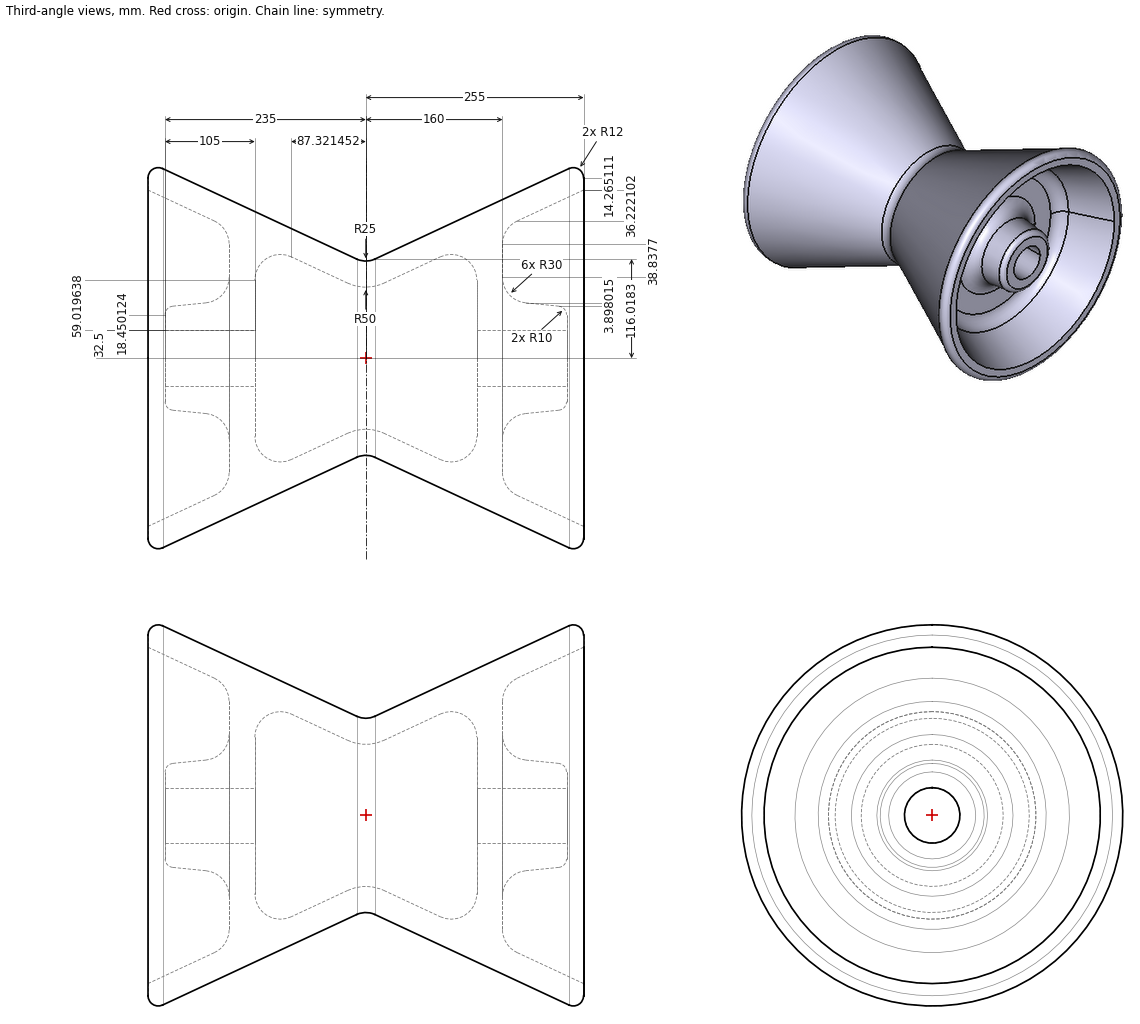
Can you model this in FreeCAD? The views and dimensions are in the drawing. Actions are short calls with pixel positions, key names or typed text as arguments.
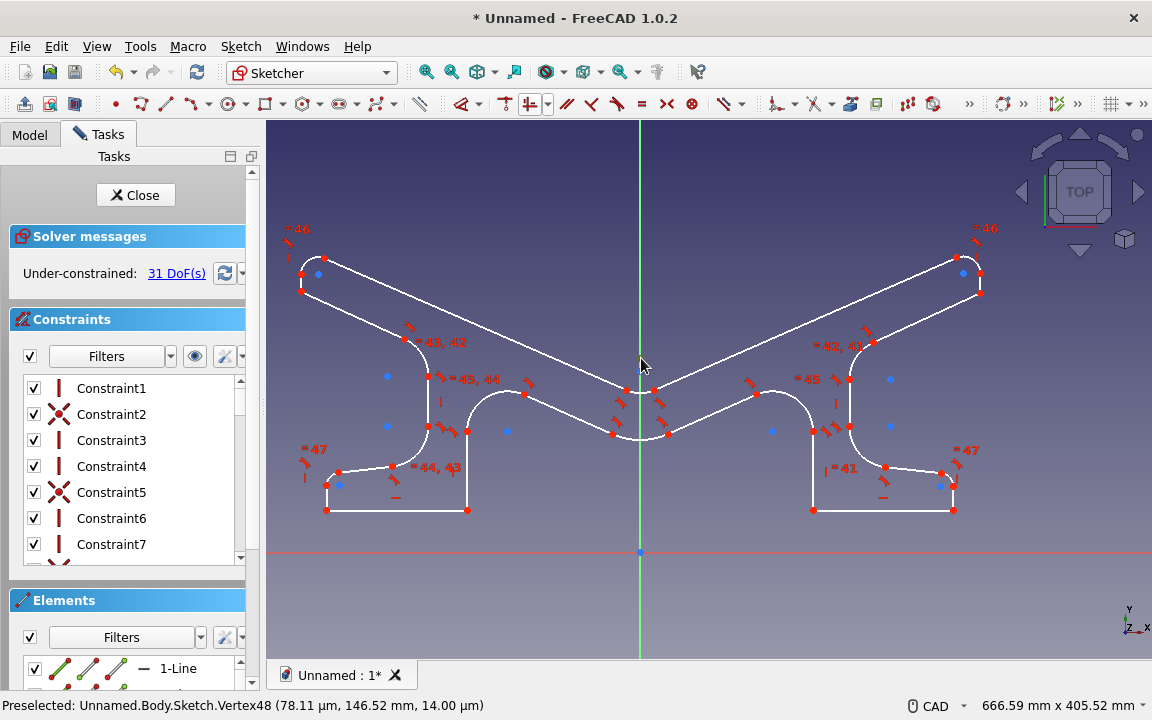
click(640, 596)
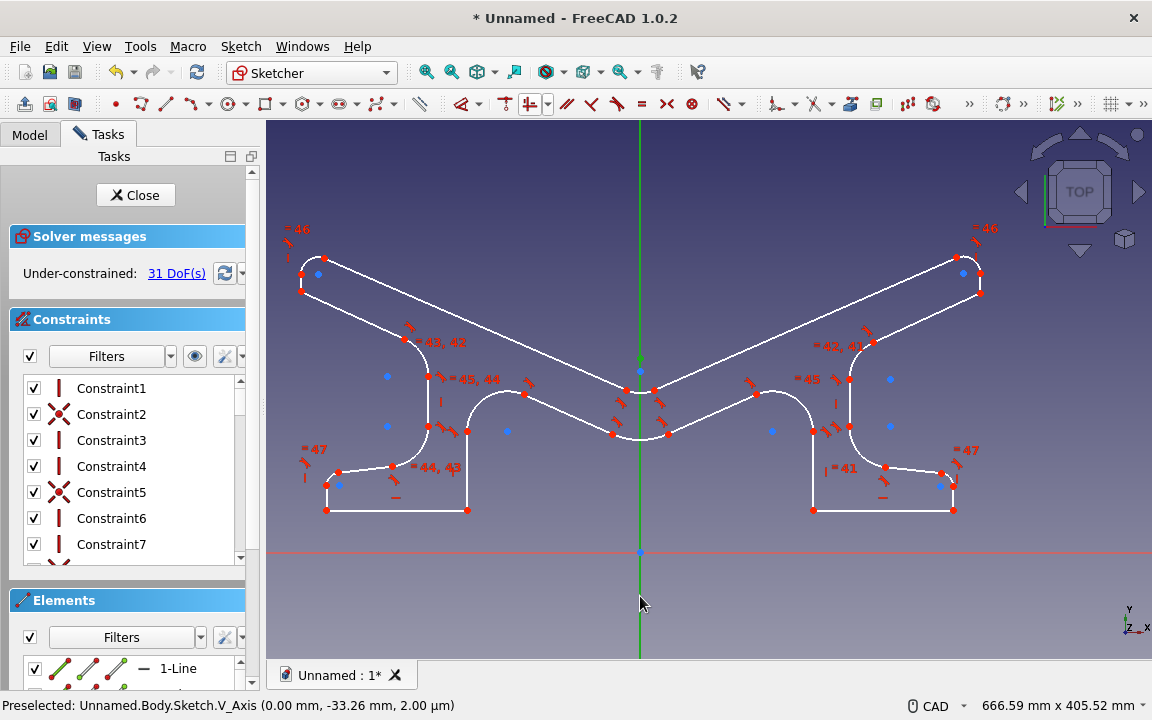
key(c)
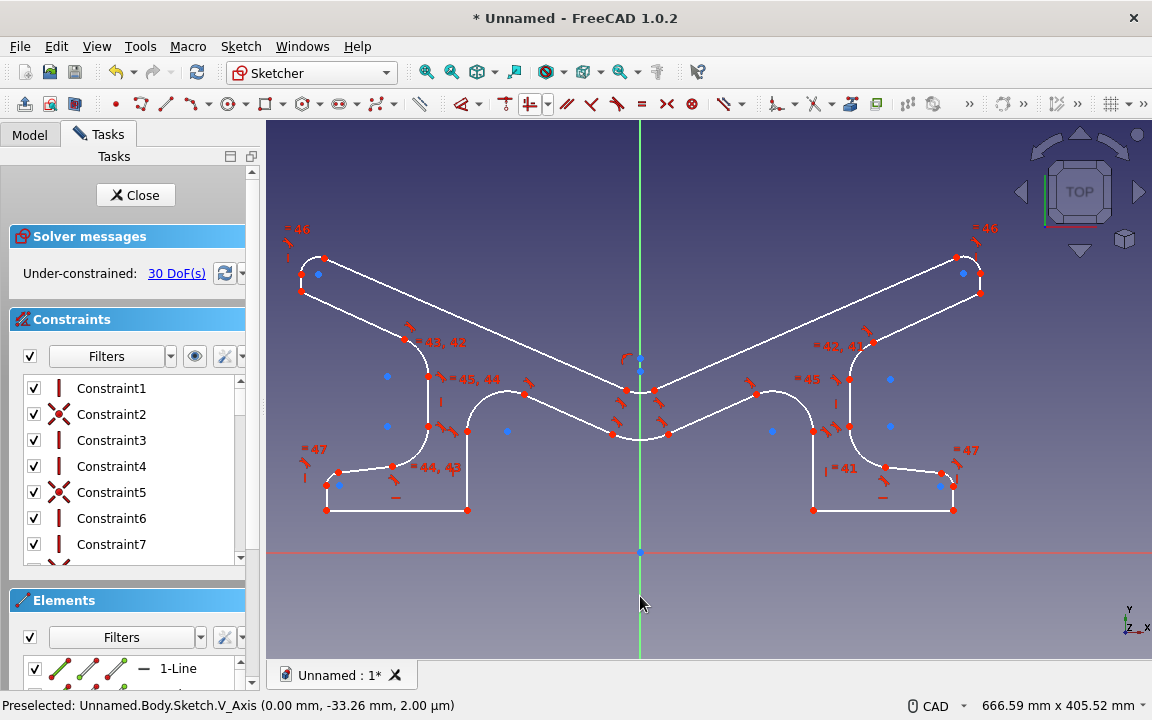
click(640, 371)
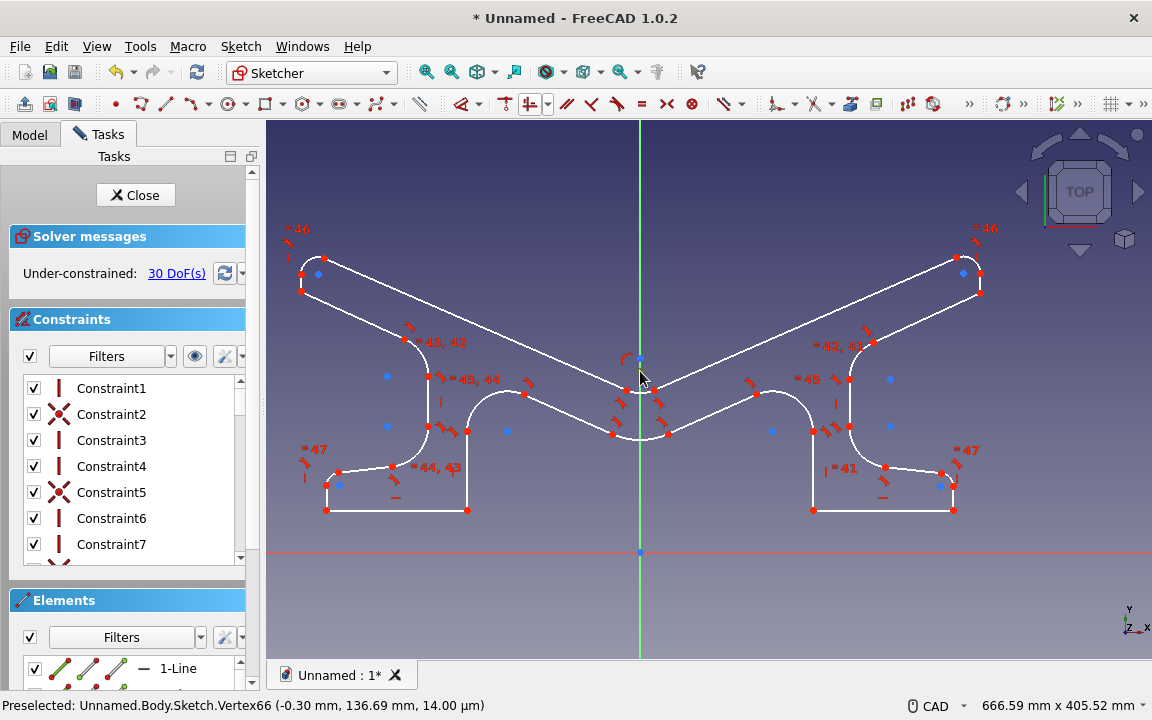
click(640, 596)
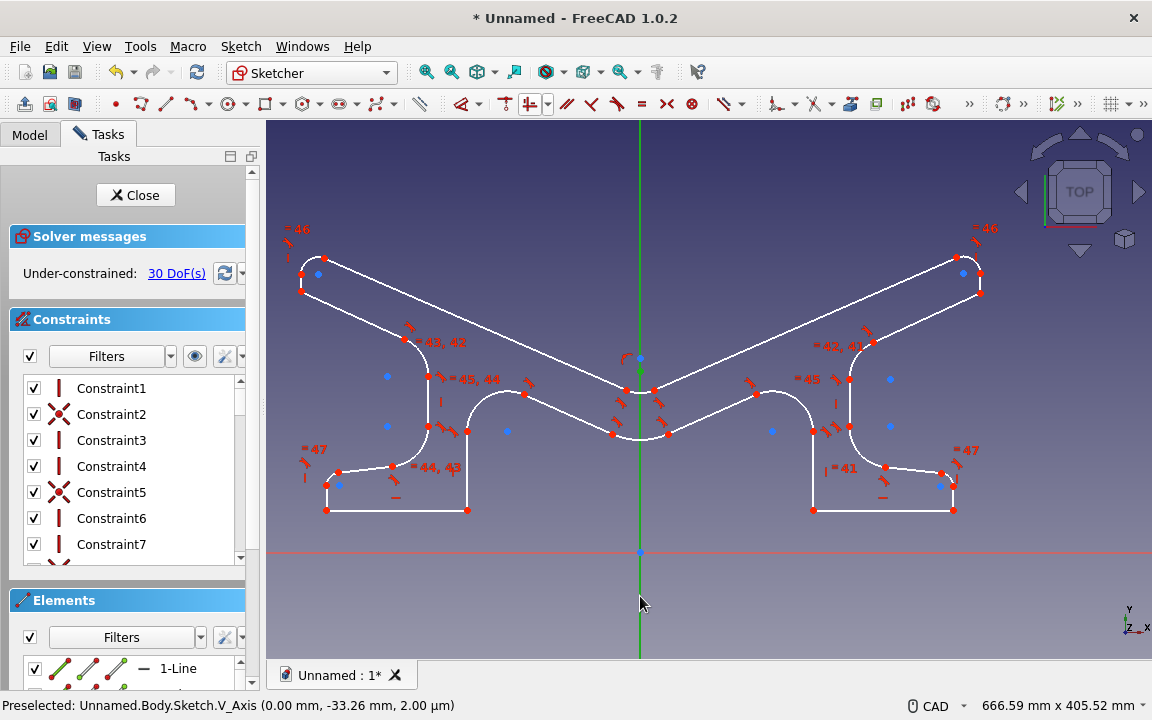
click(505, 104)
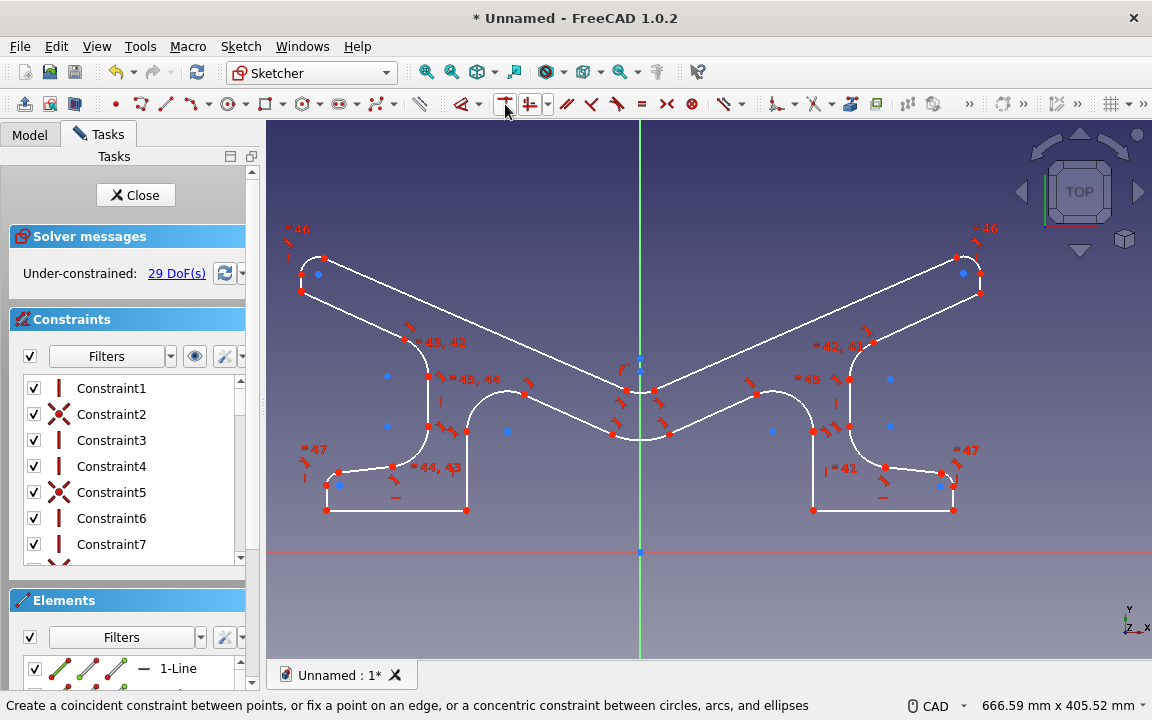
click(963, 273)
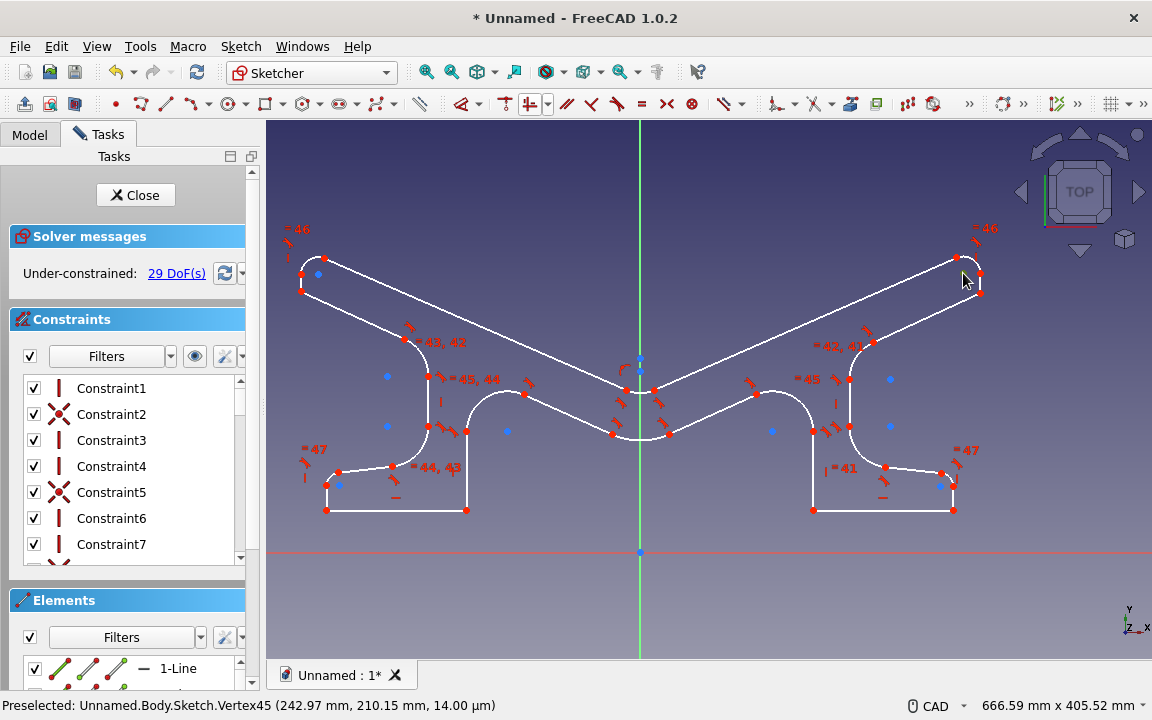
click(318, 274)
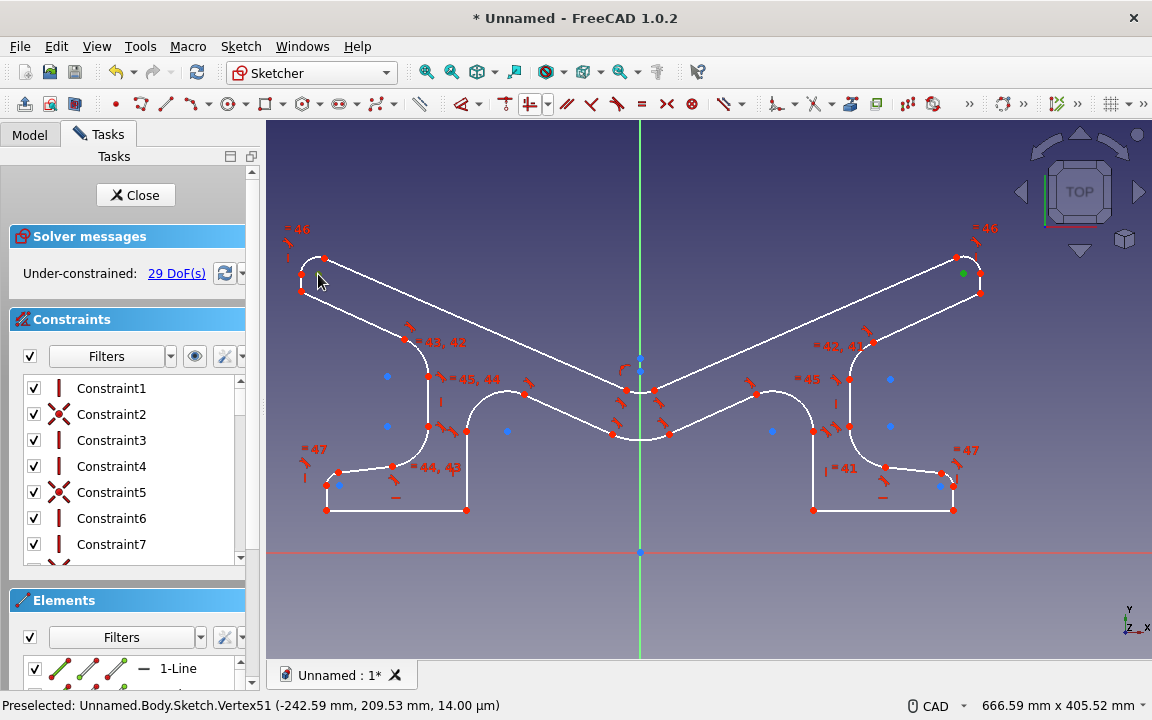
click(640, 596)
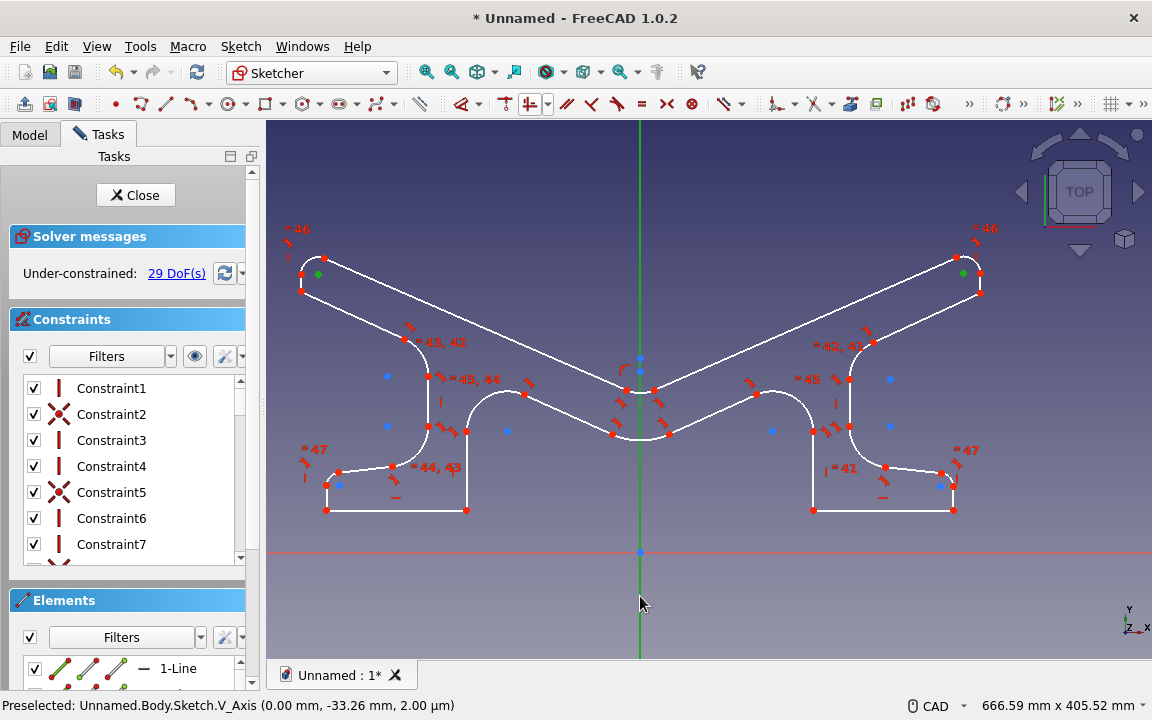
click(667, 104)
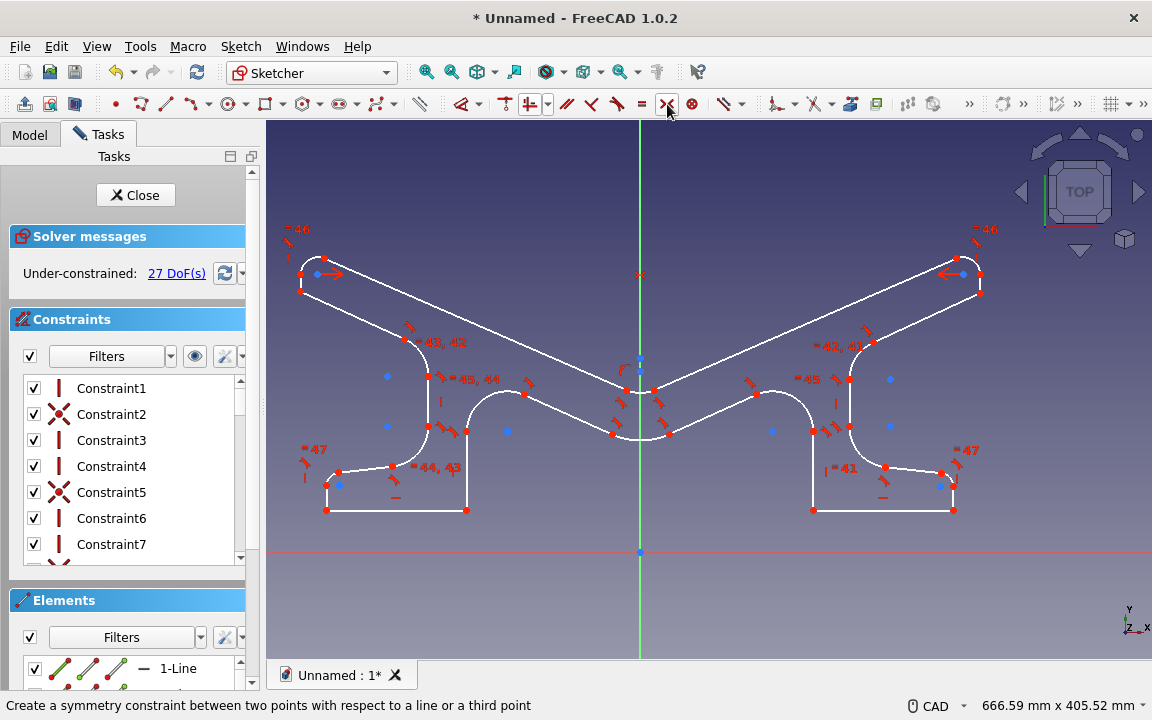
click(890, 379)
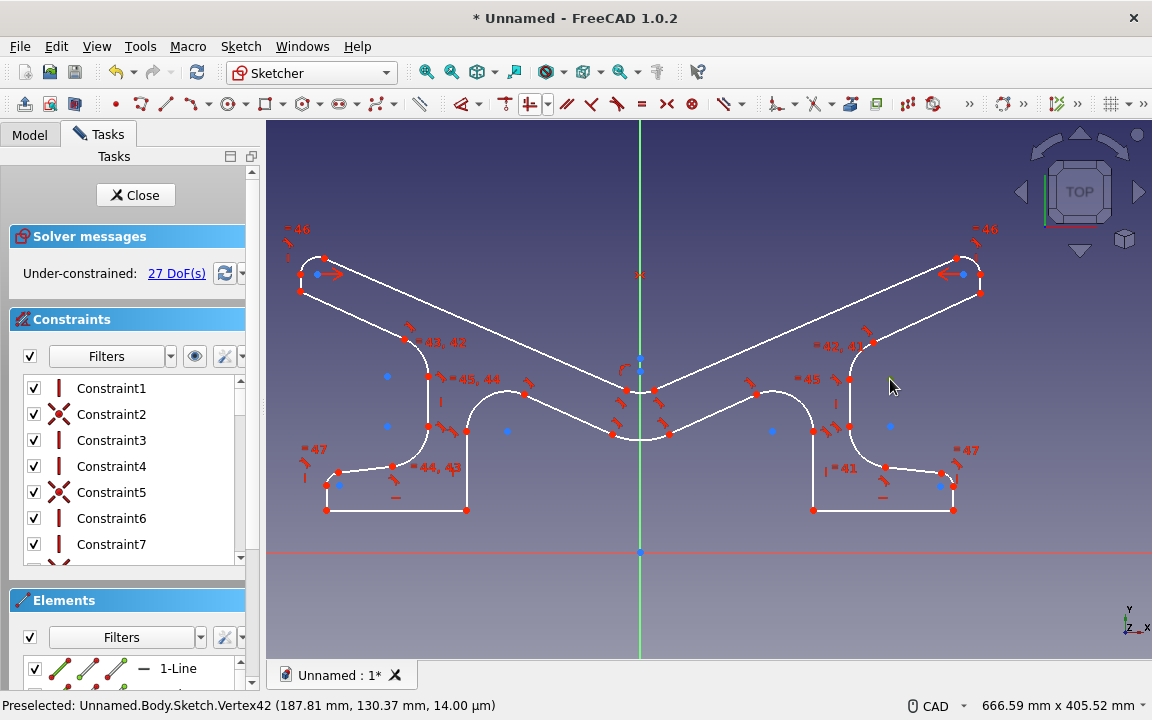
click(388, 376)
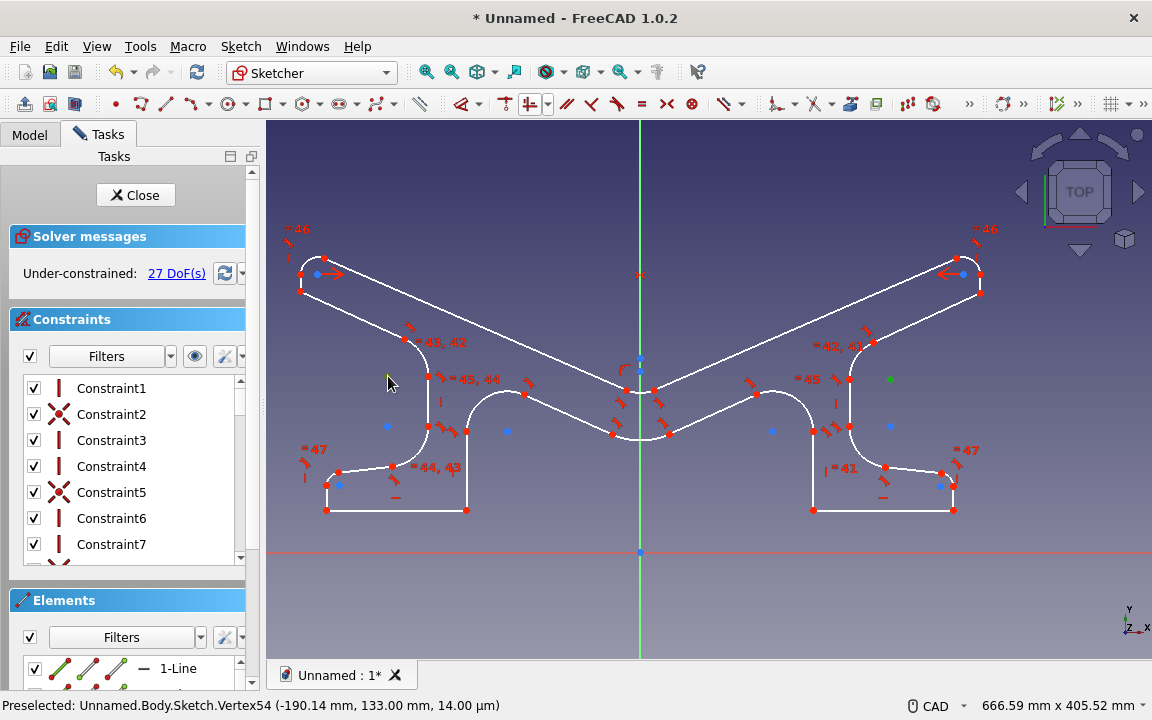
click(640, 596)